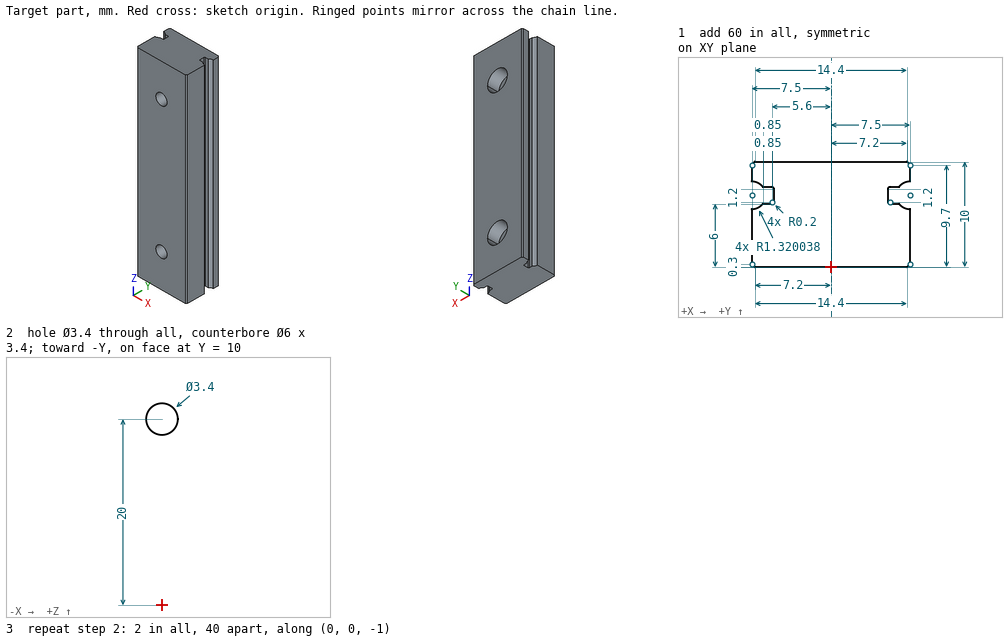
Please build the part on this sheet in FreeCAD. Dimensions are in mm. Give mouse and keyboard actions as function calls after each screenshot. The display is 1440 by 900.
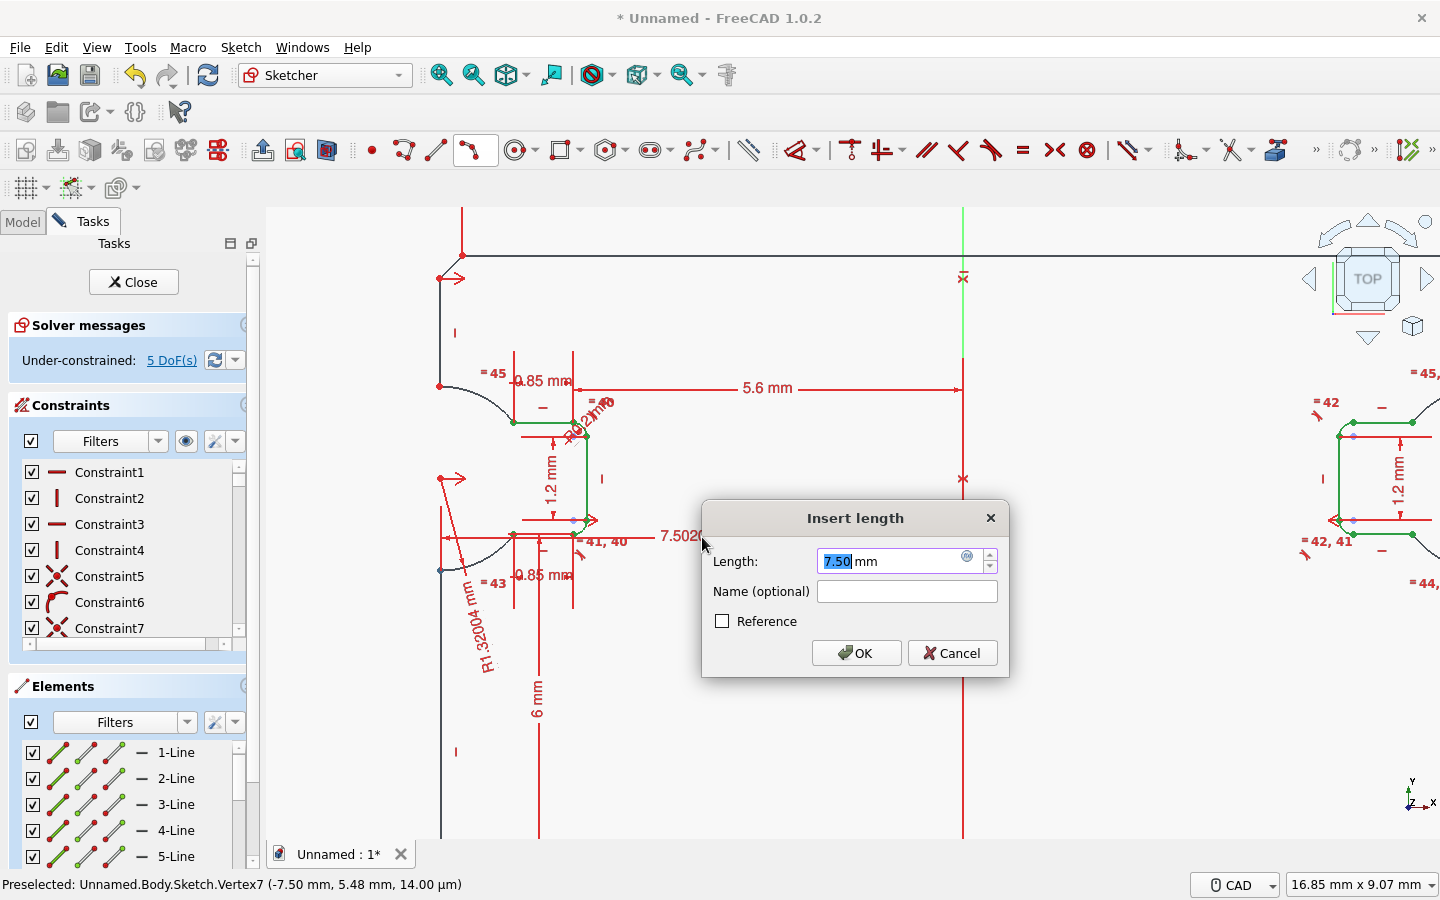
text(7.5)
key(Return)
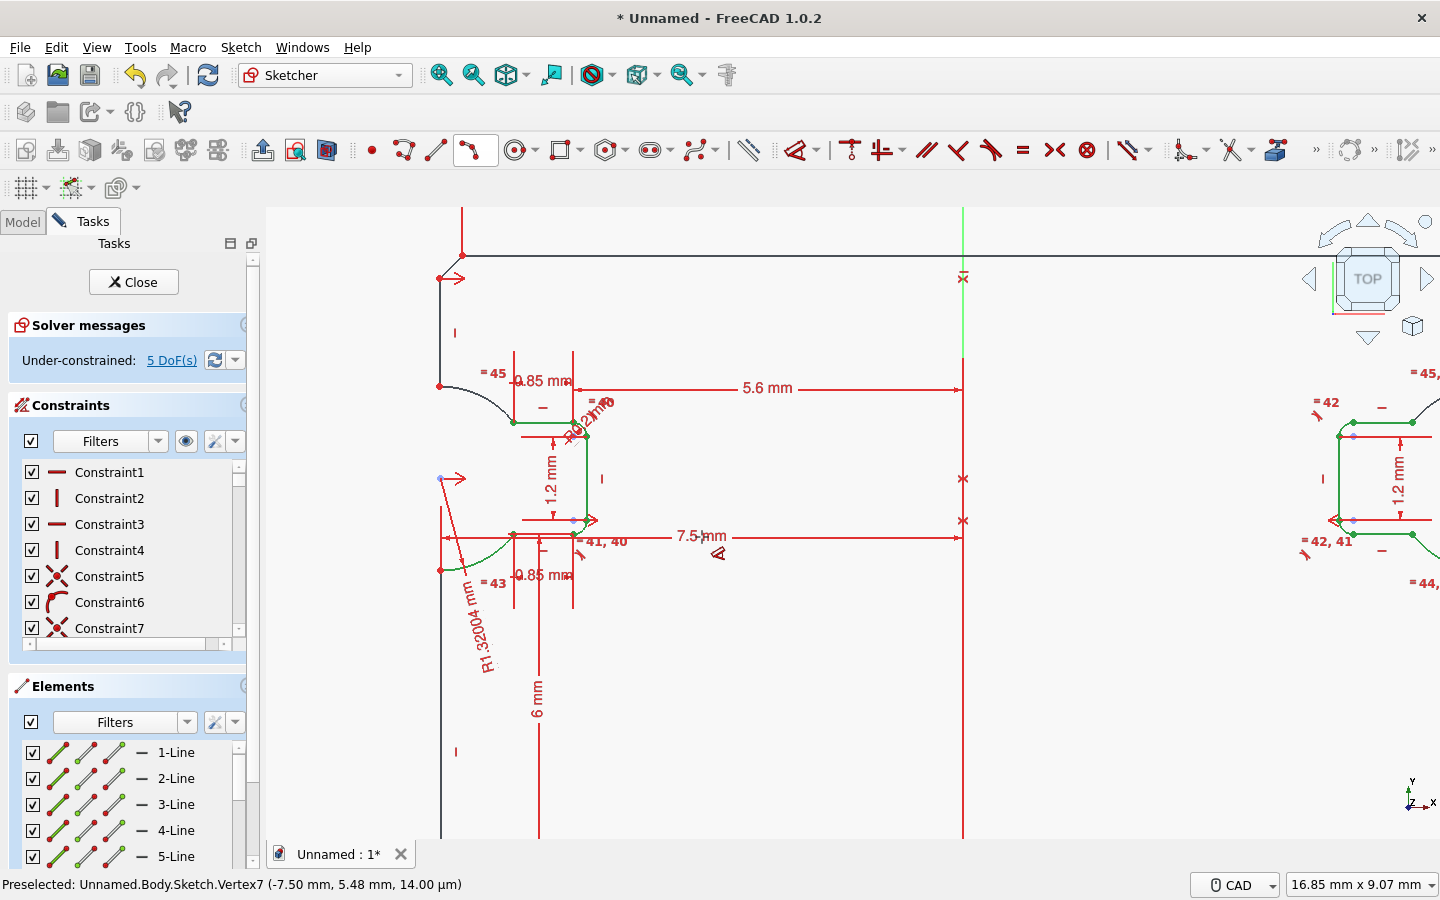
scroll(567, 424, down, 3)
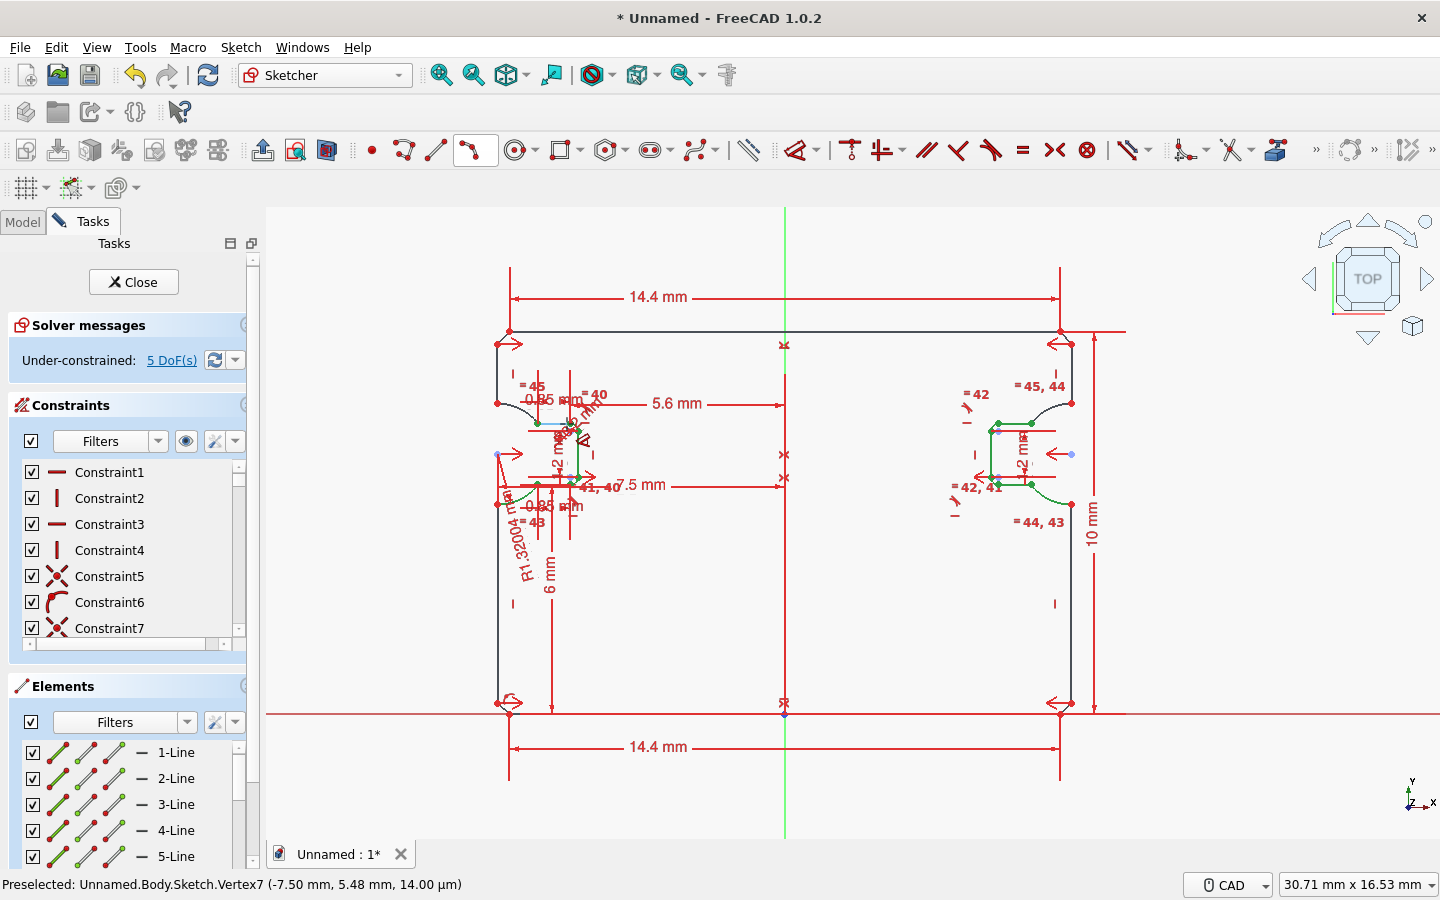
scroll(498, 703, up, 7)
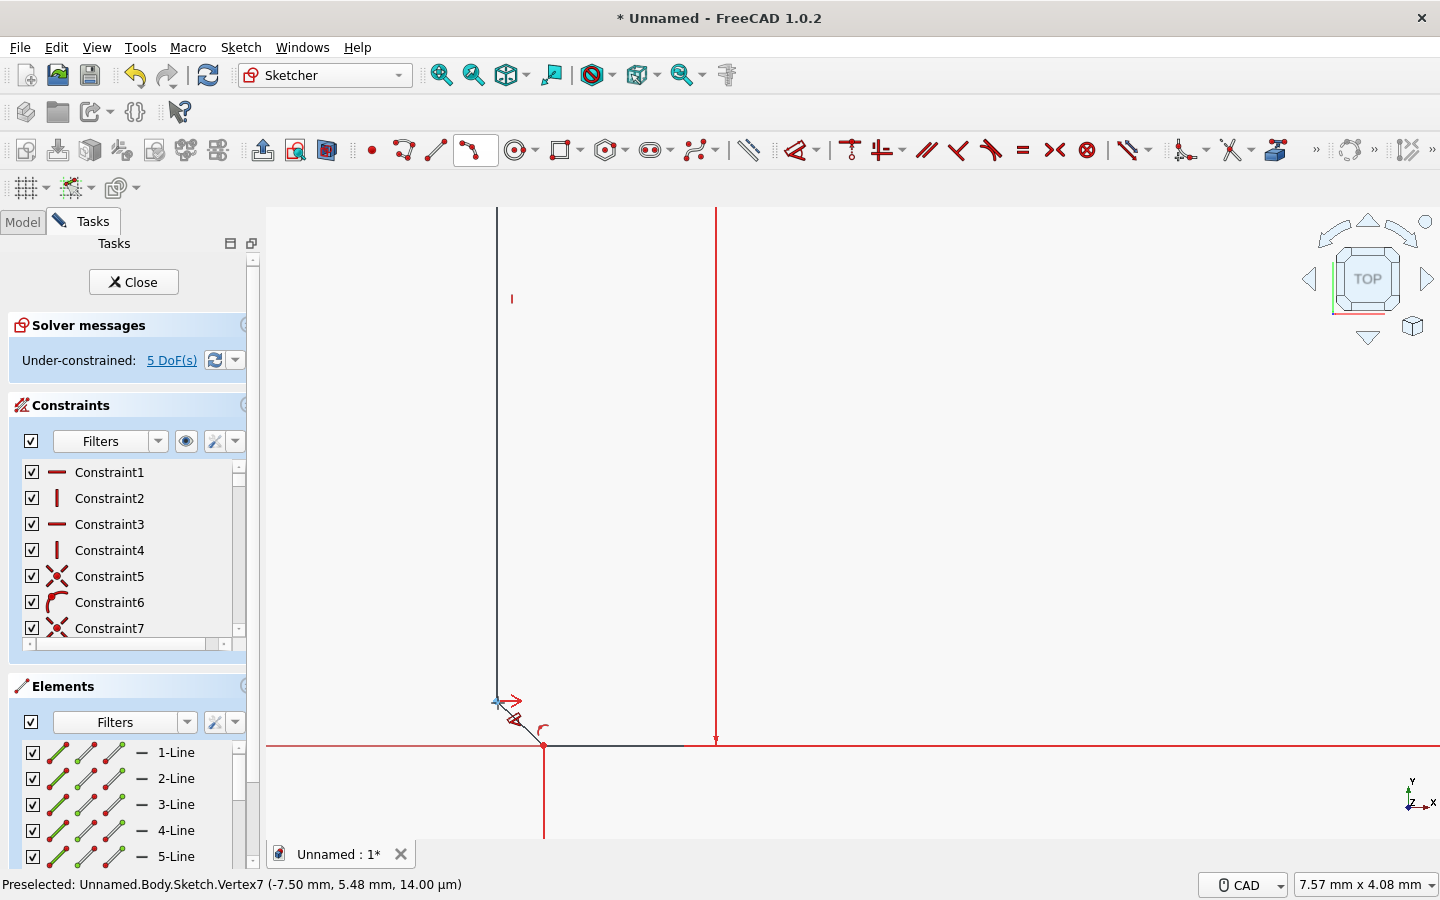
click(497, 701)
click(463, 723)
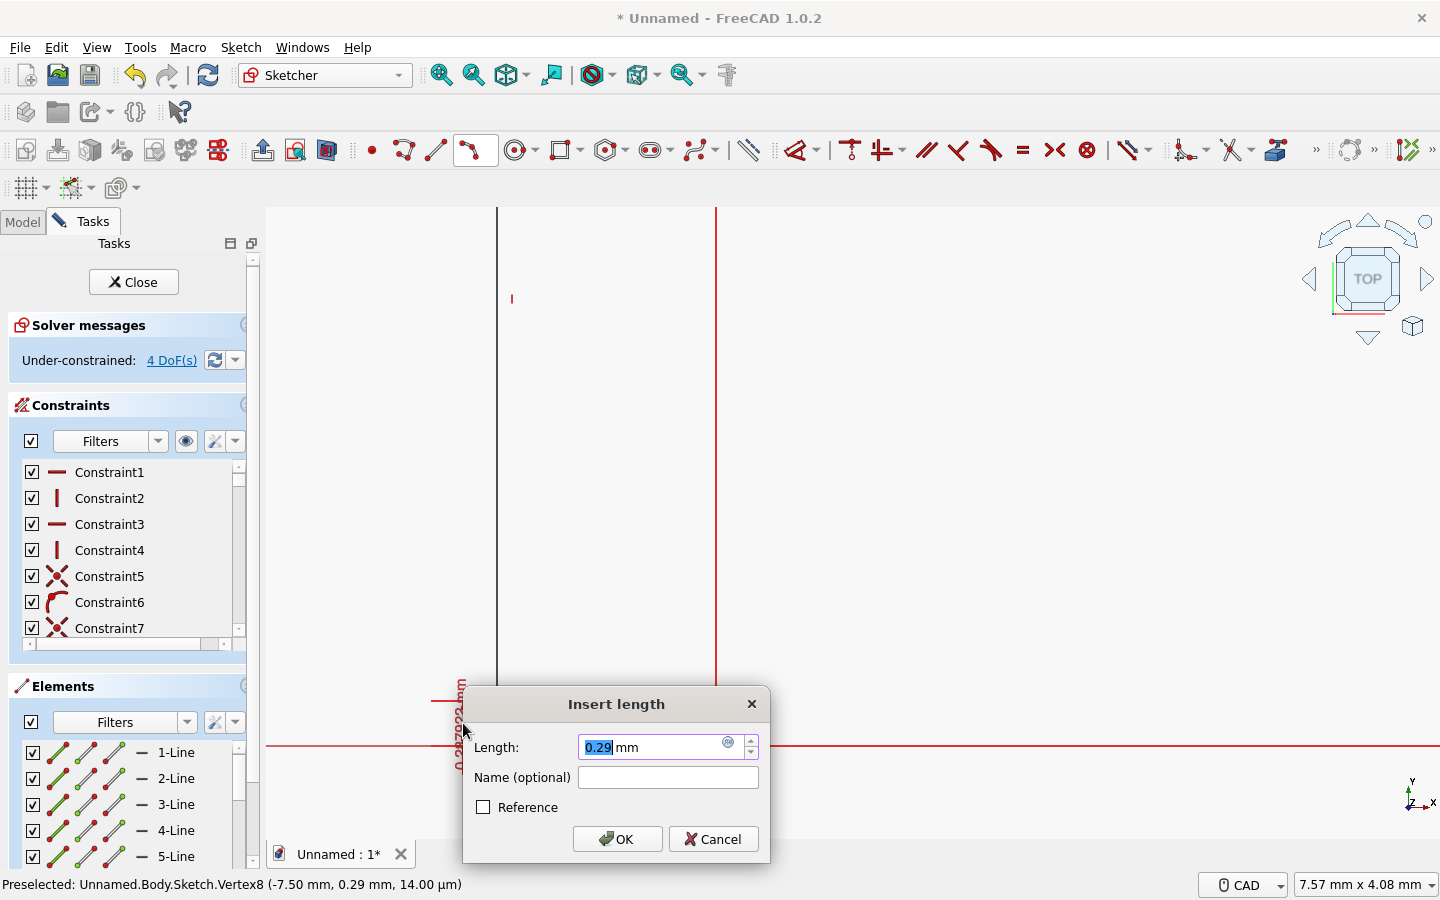
text(0.3)
key(Return)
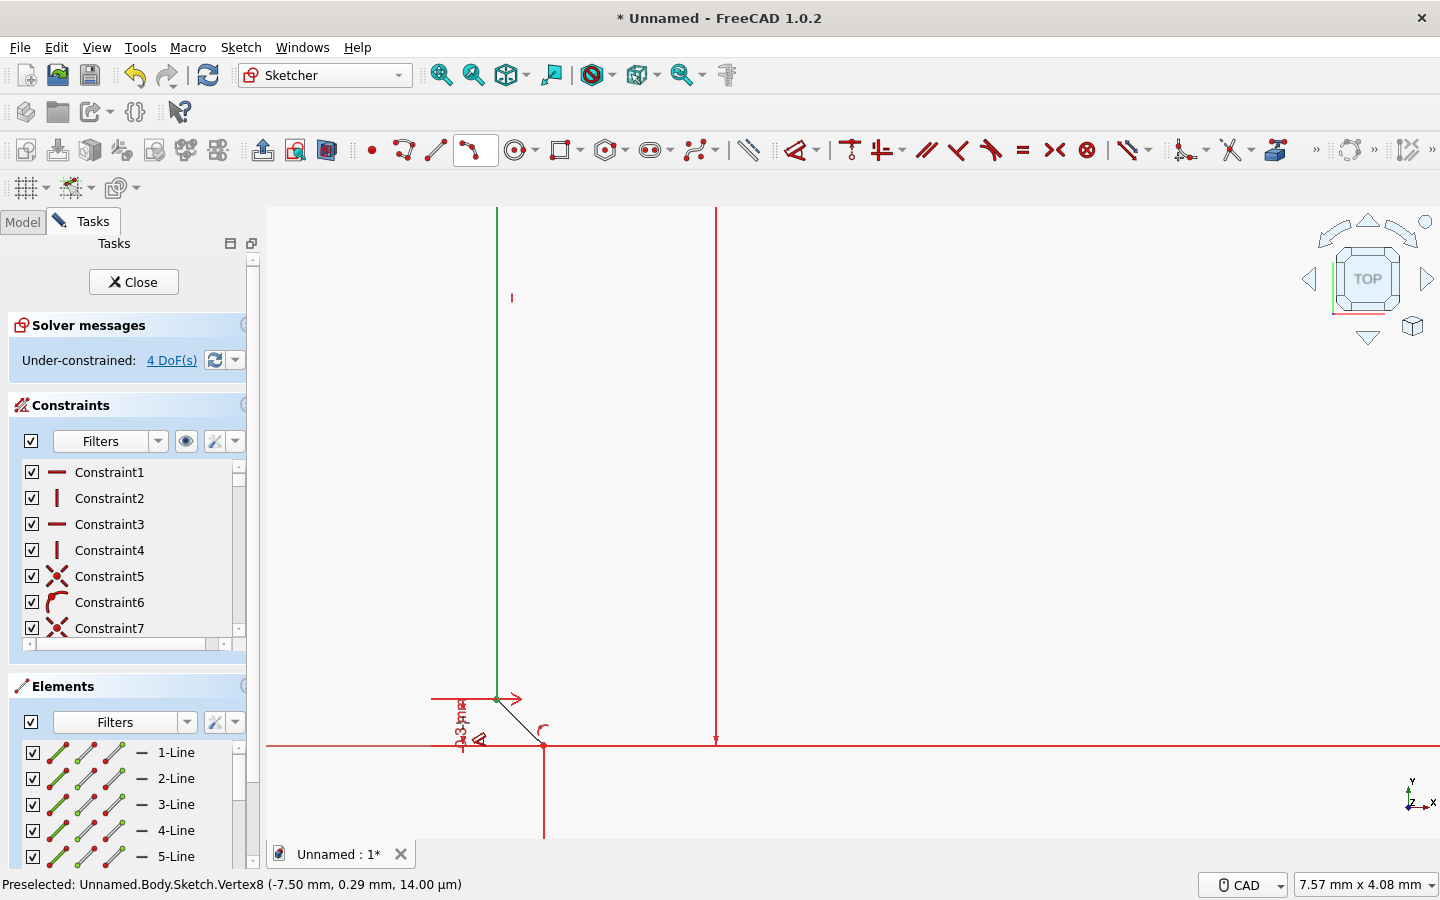
scroll(498, 704, down, 7)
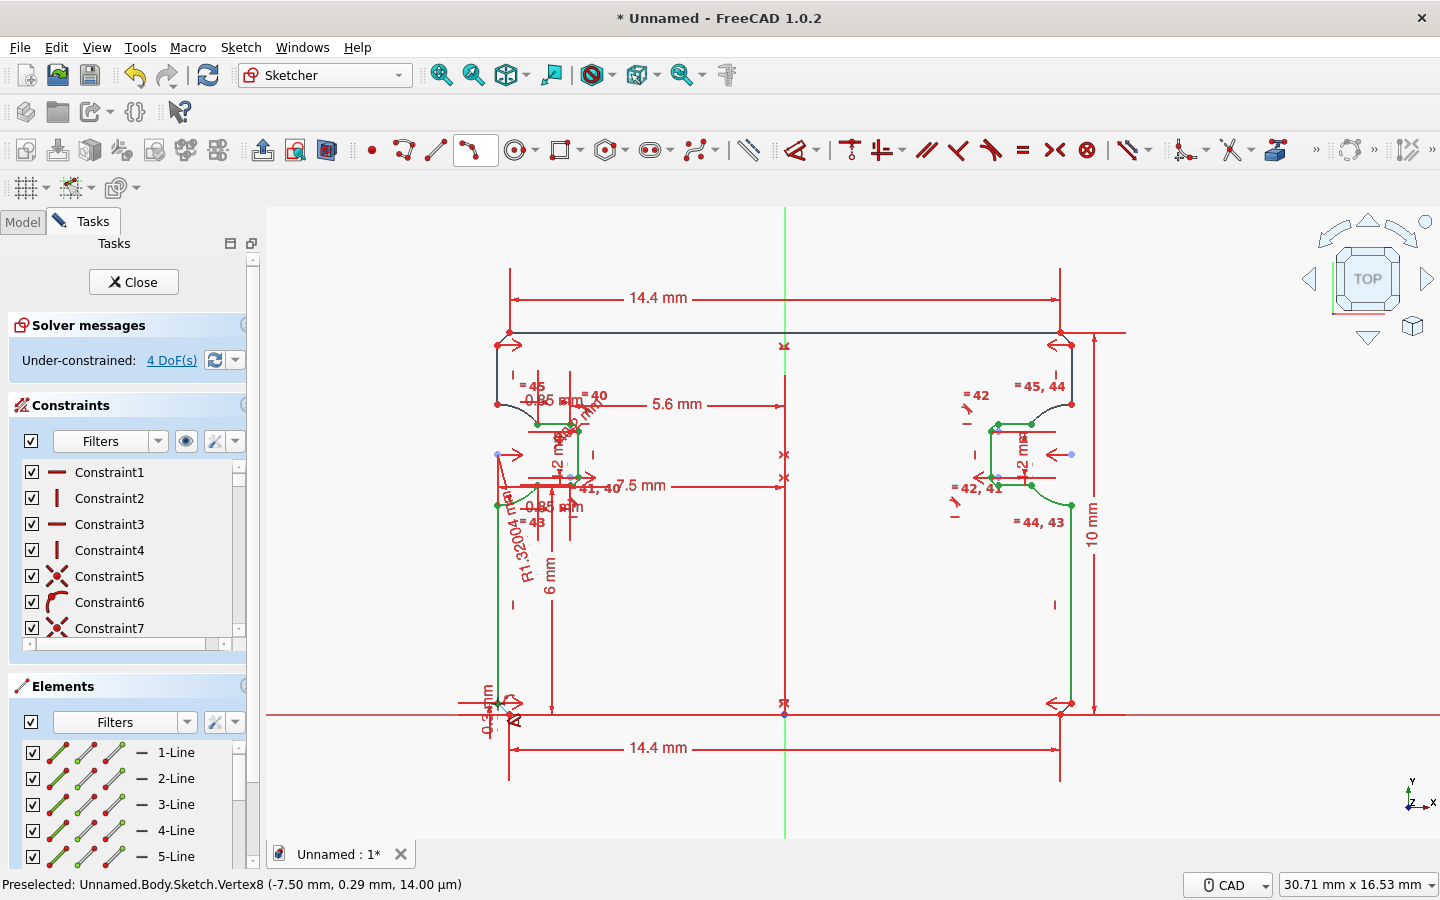
click(509, 715)
click(584, 749)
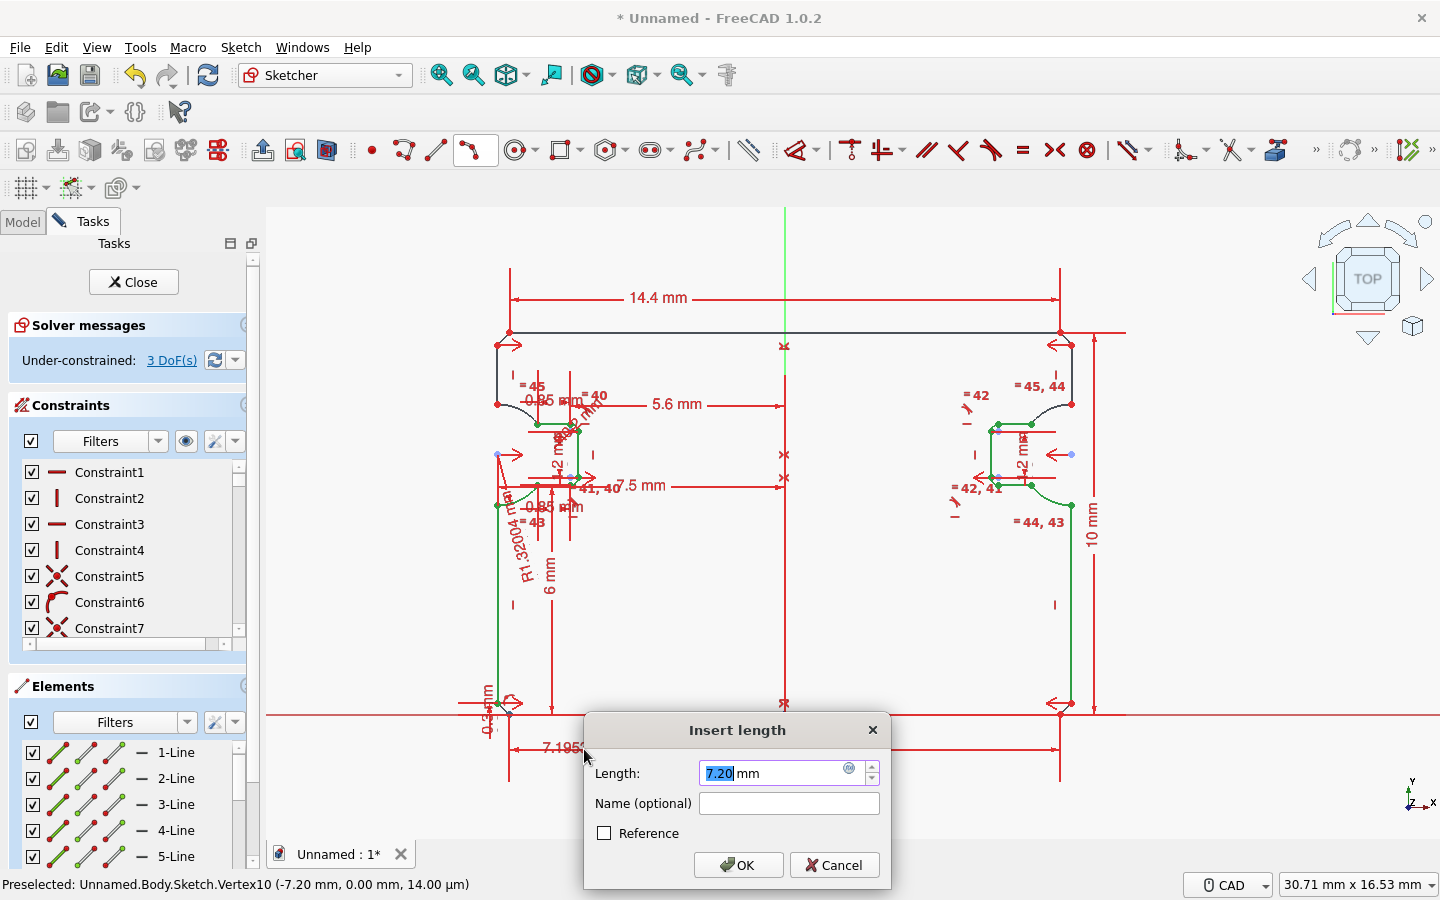
text(7.2)
key(Return)